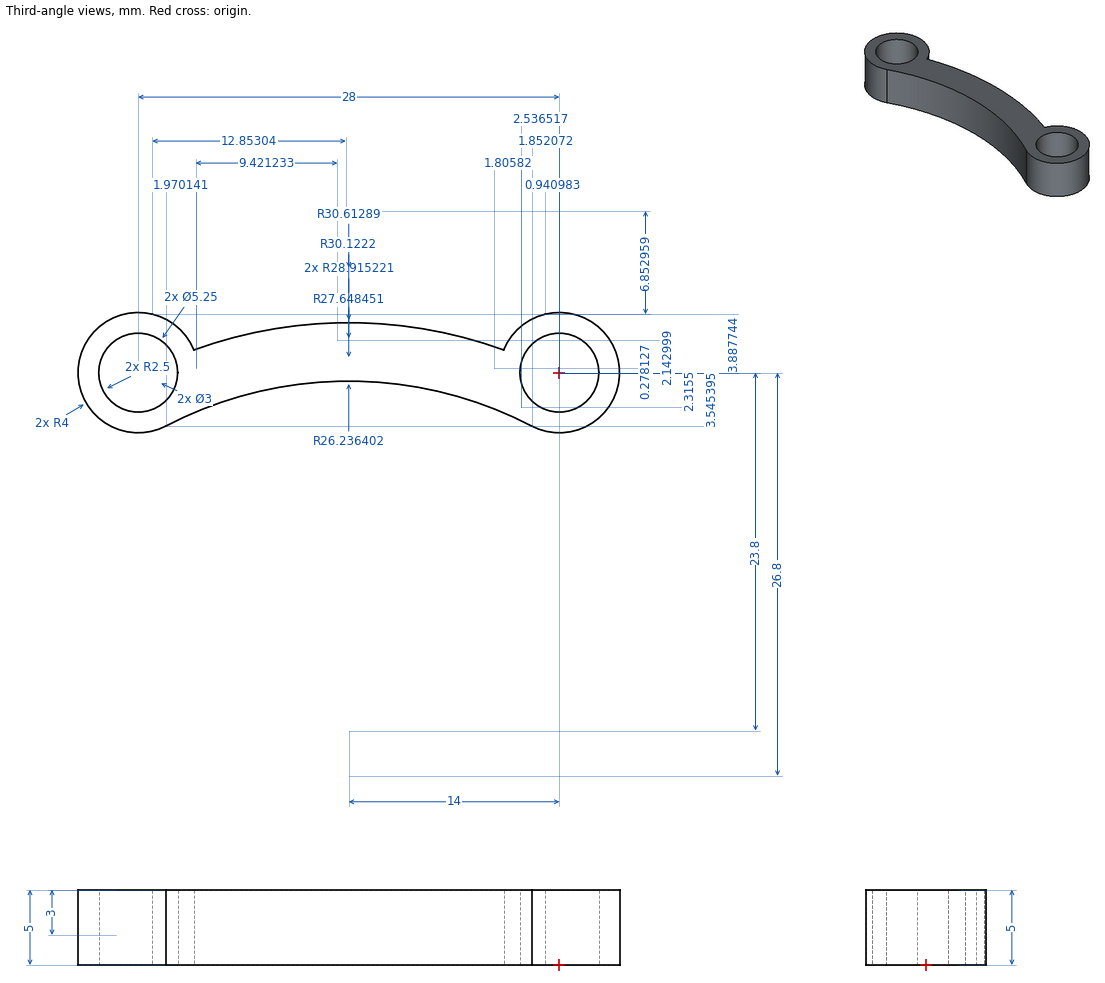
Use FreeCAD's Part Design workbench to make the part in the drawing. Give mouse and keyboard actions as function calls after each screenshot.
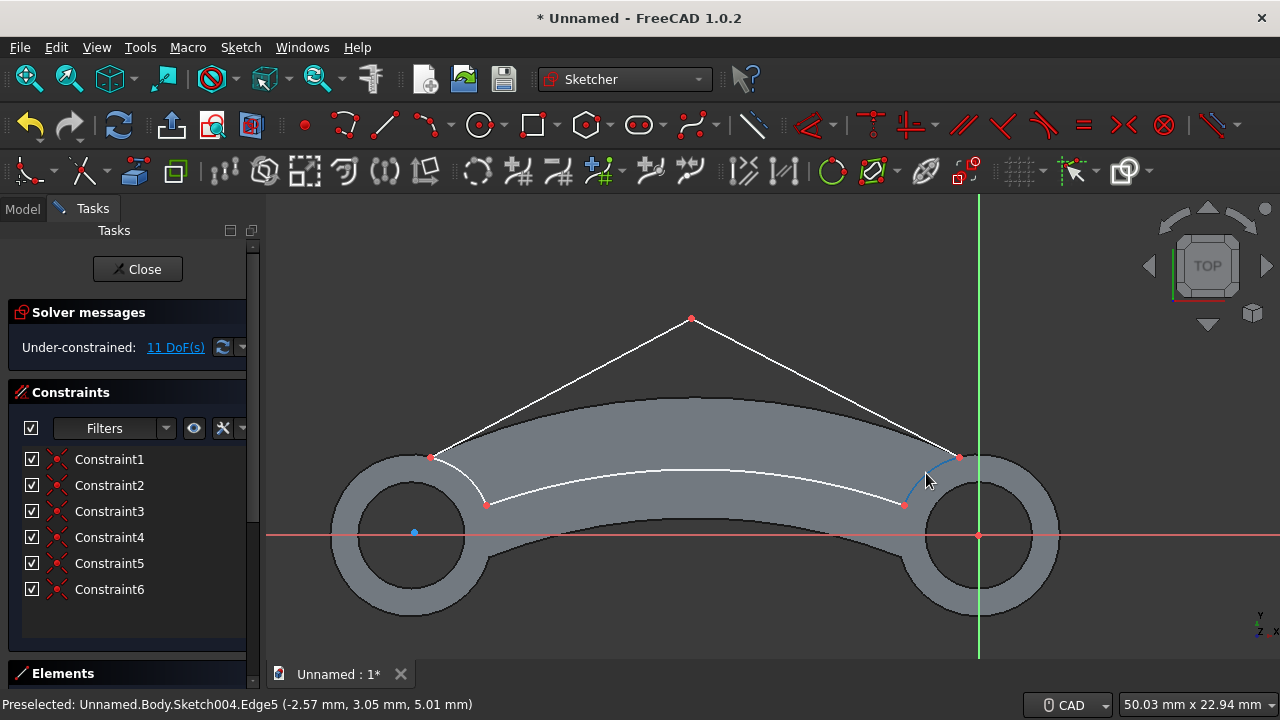
click(475, 486)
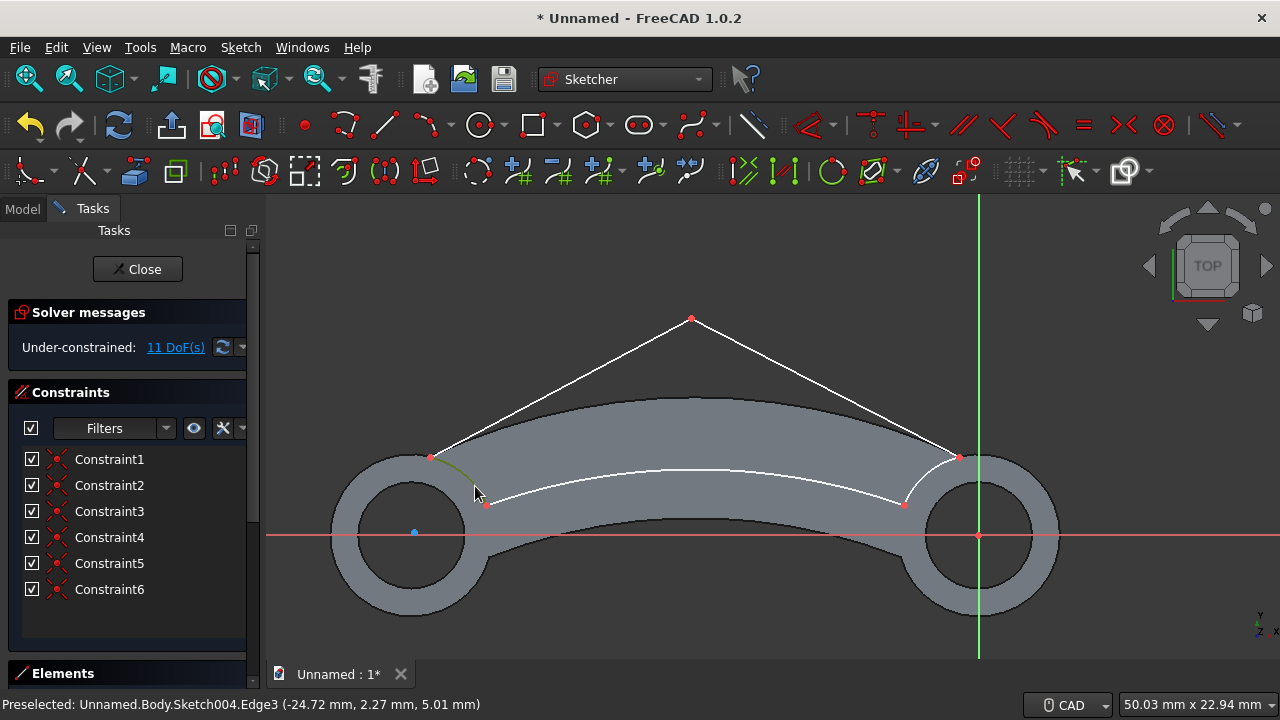
click(938, 466)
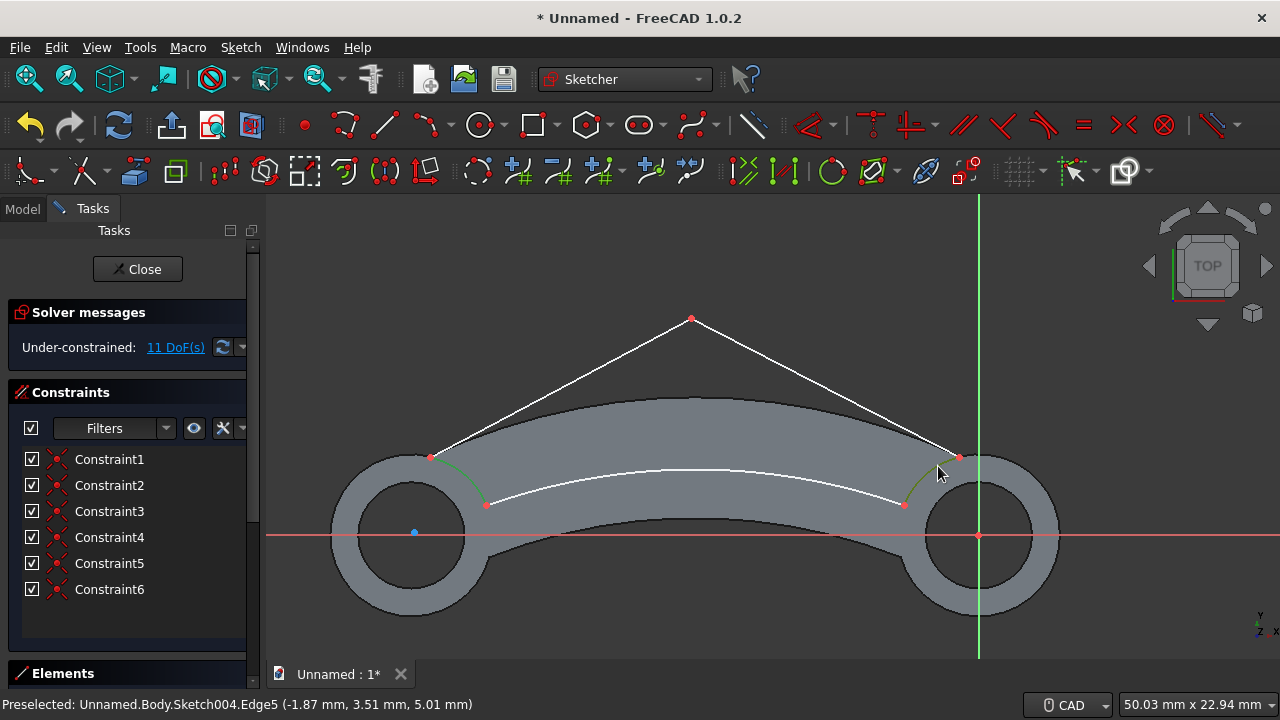
click(1084, 126)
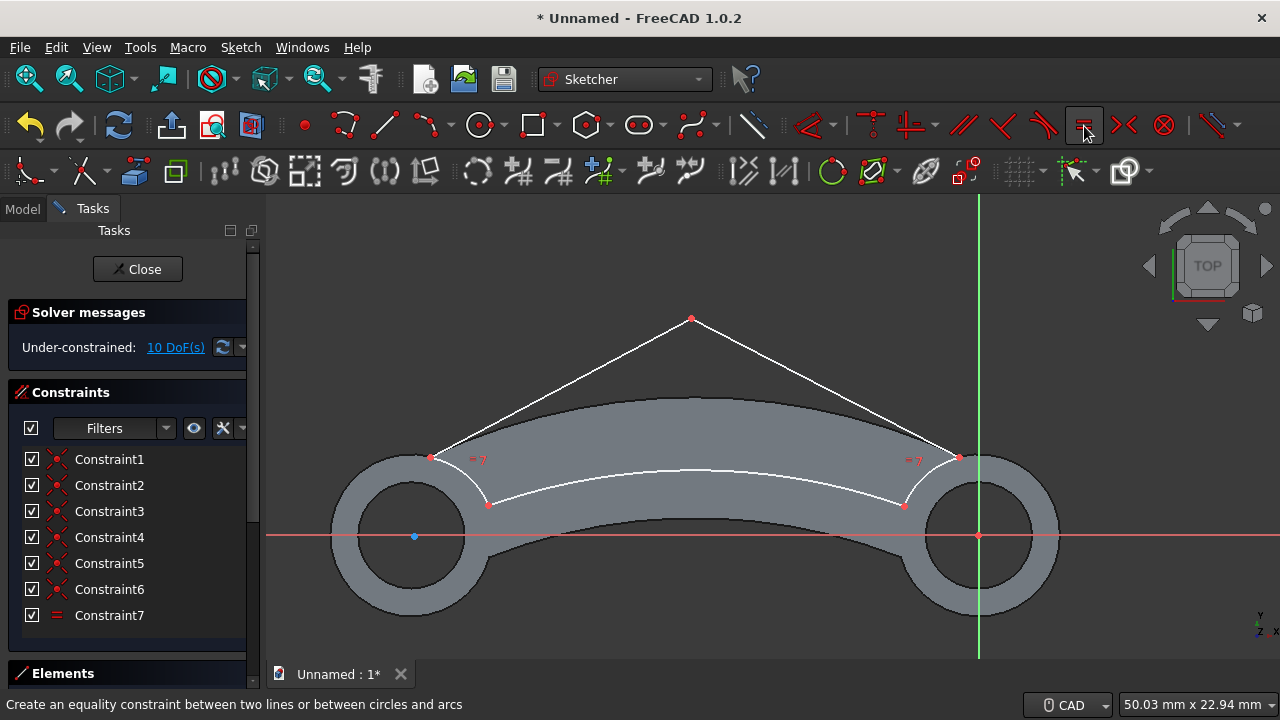
click(415, 536)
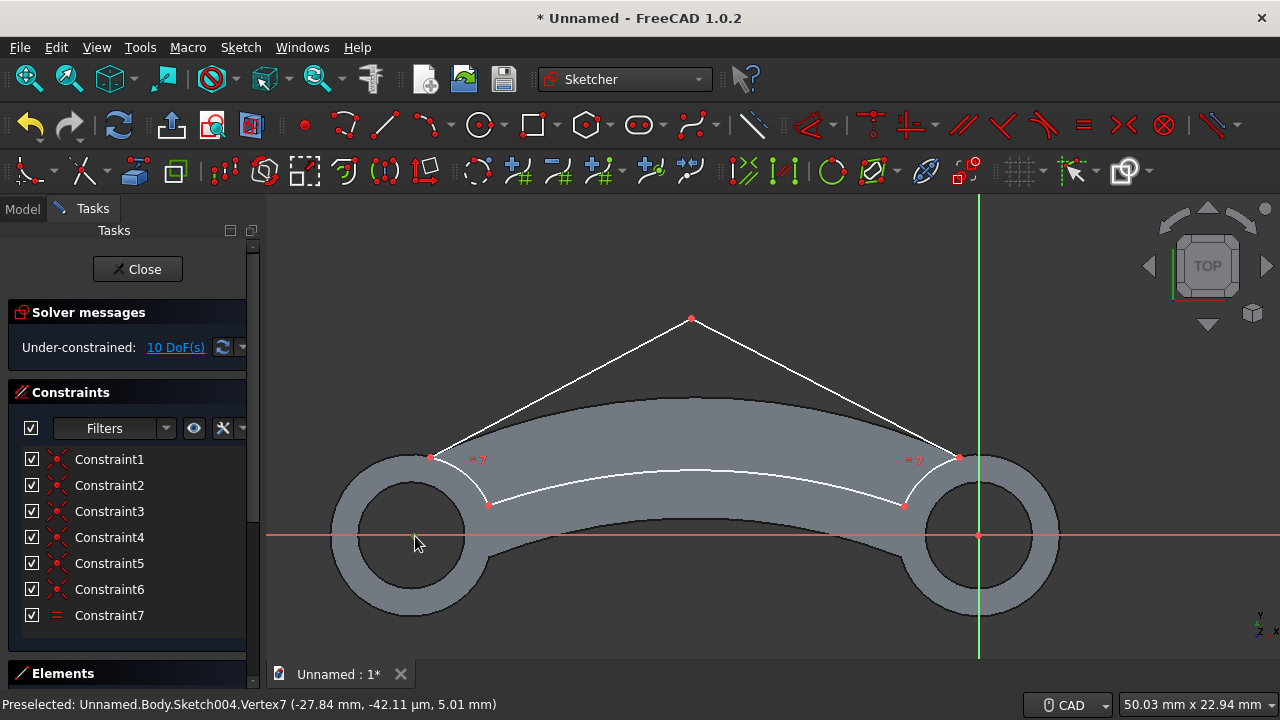
click(353, 535)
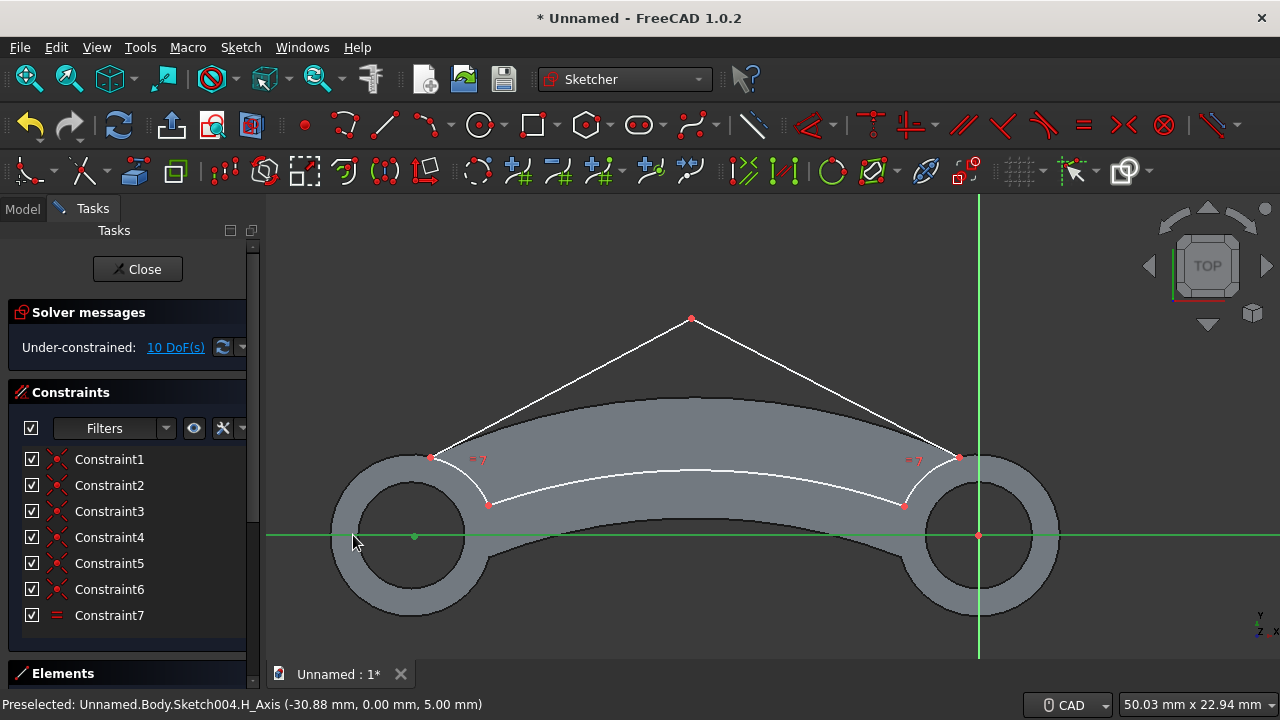
key(c)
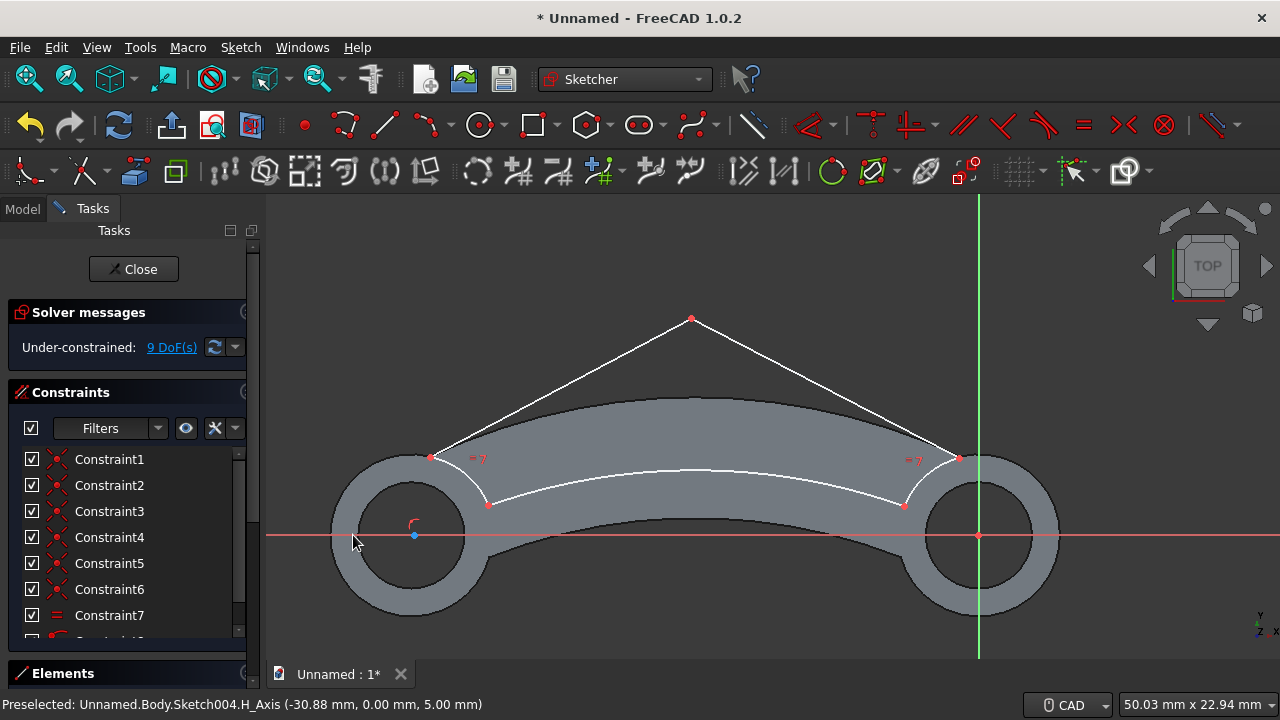
click(808, 126)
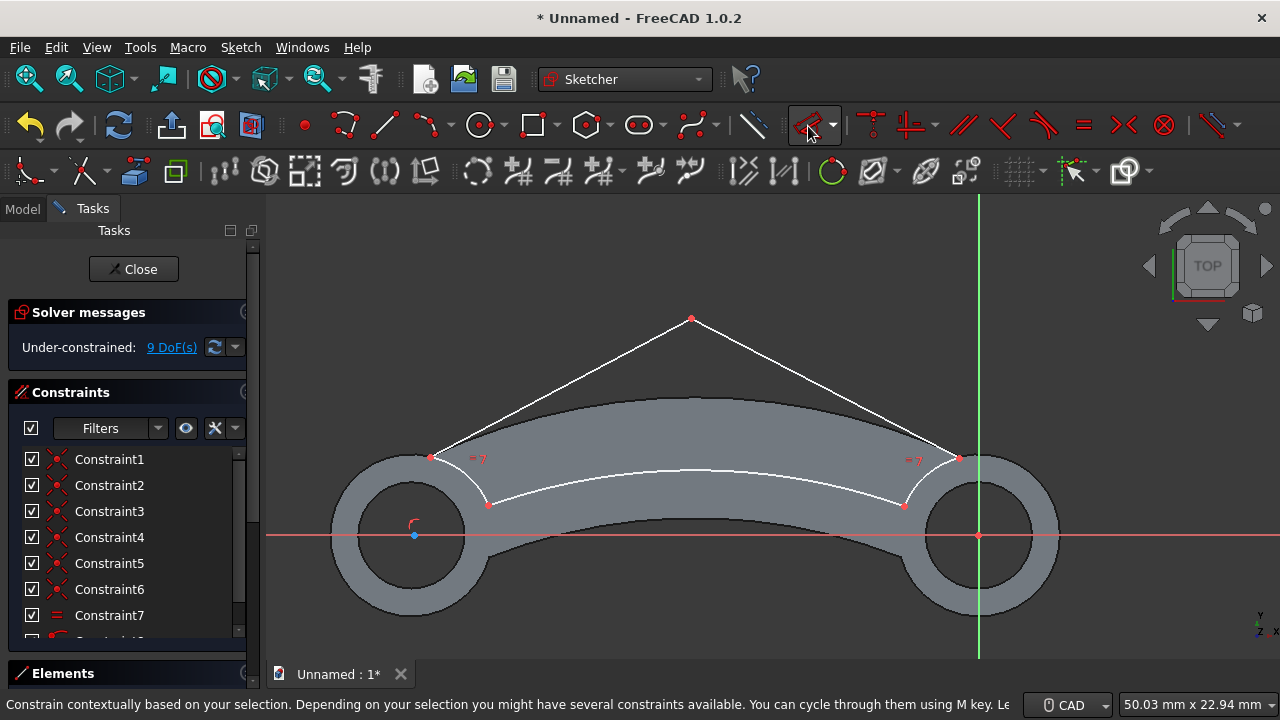
click(477, 485)
click(502, 465)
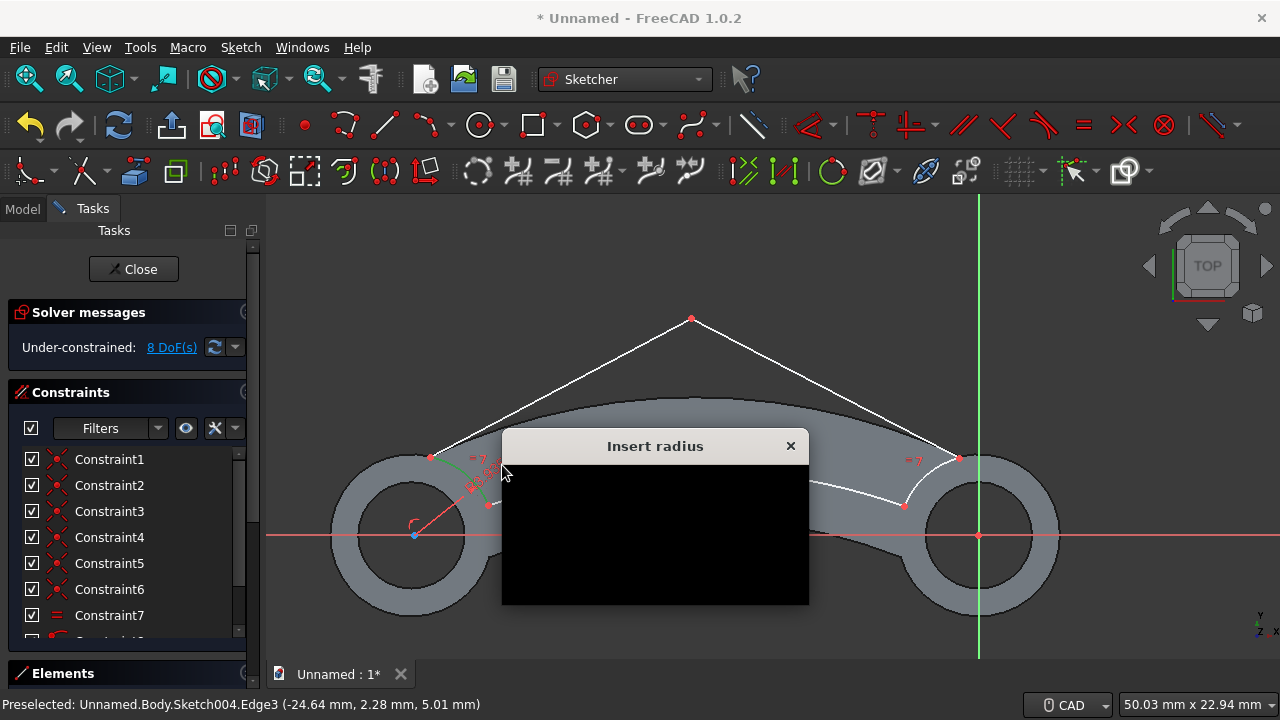
text(4)
key(Return)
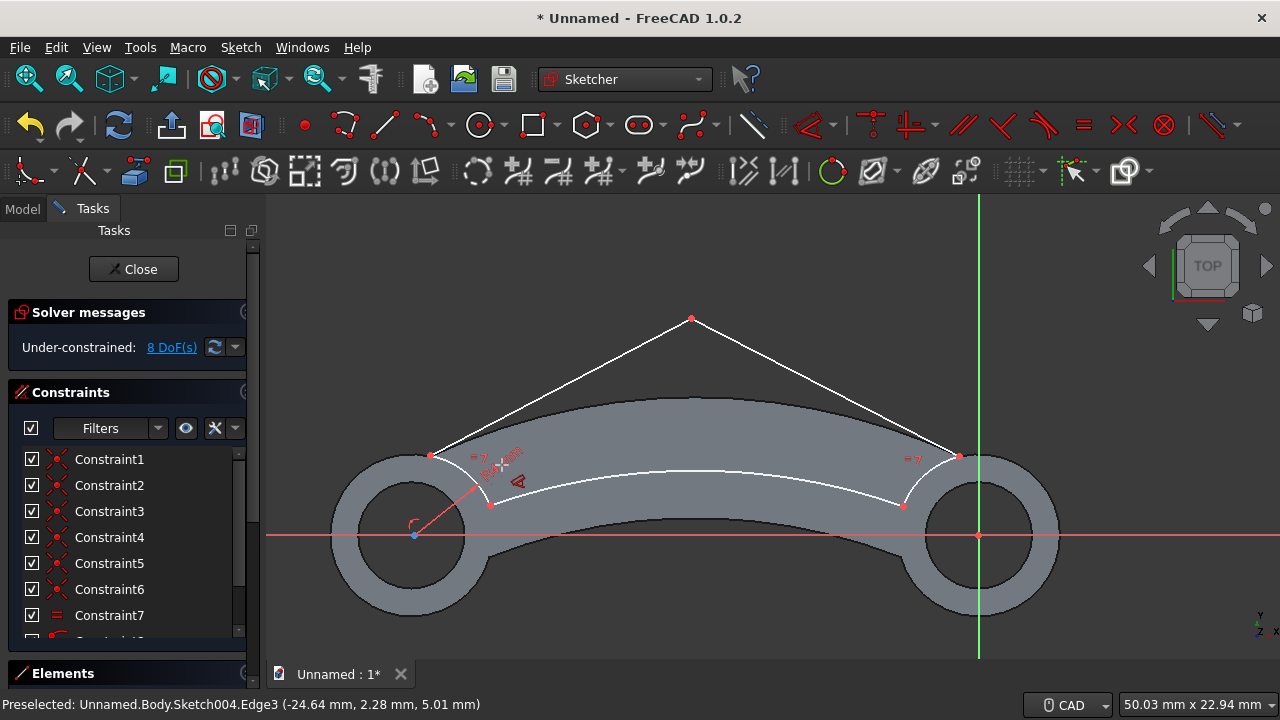
click(781, 477)
click(785, 445)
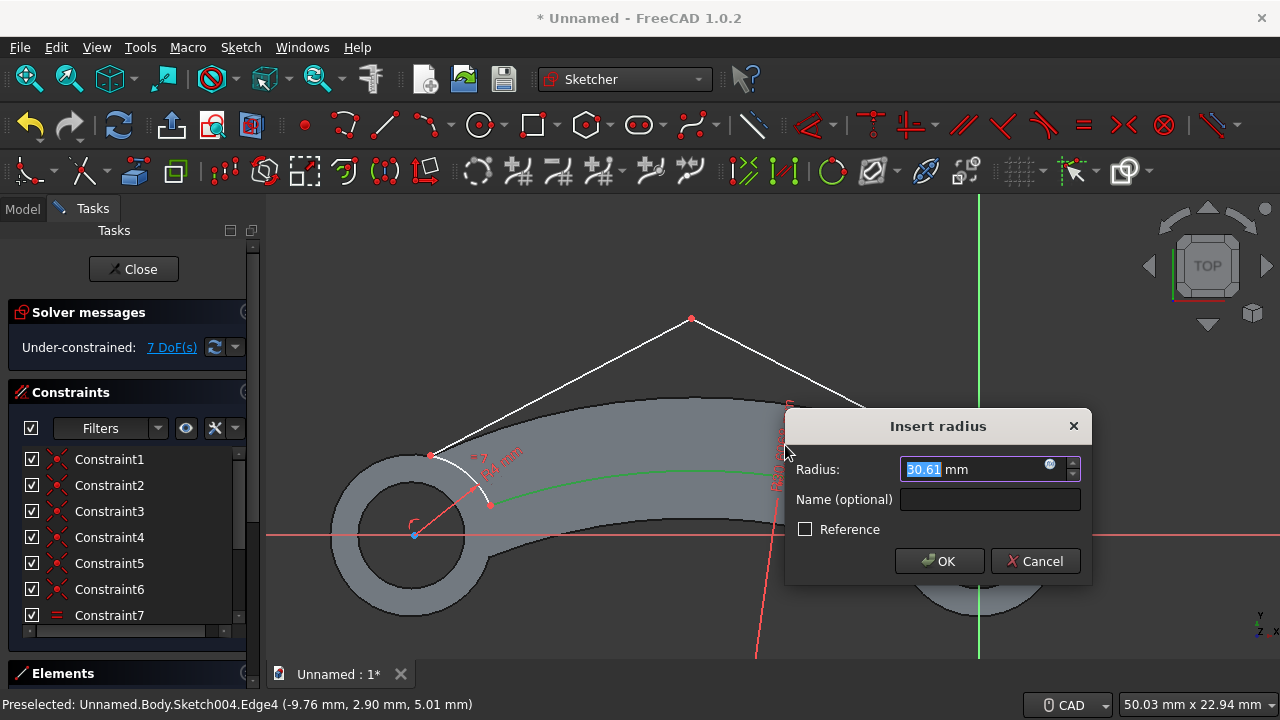
text(30.1222)
key(Return)